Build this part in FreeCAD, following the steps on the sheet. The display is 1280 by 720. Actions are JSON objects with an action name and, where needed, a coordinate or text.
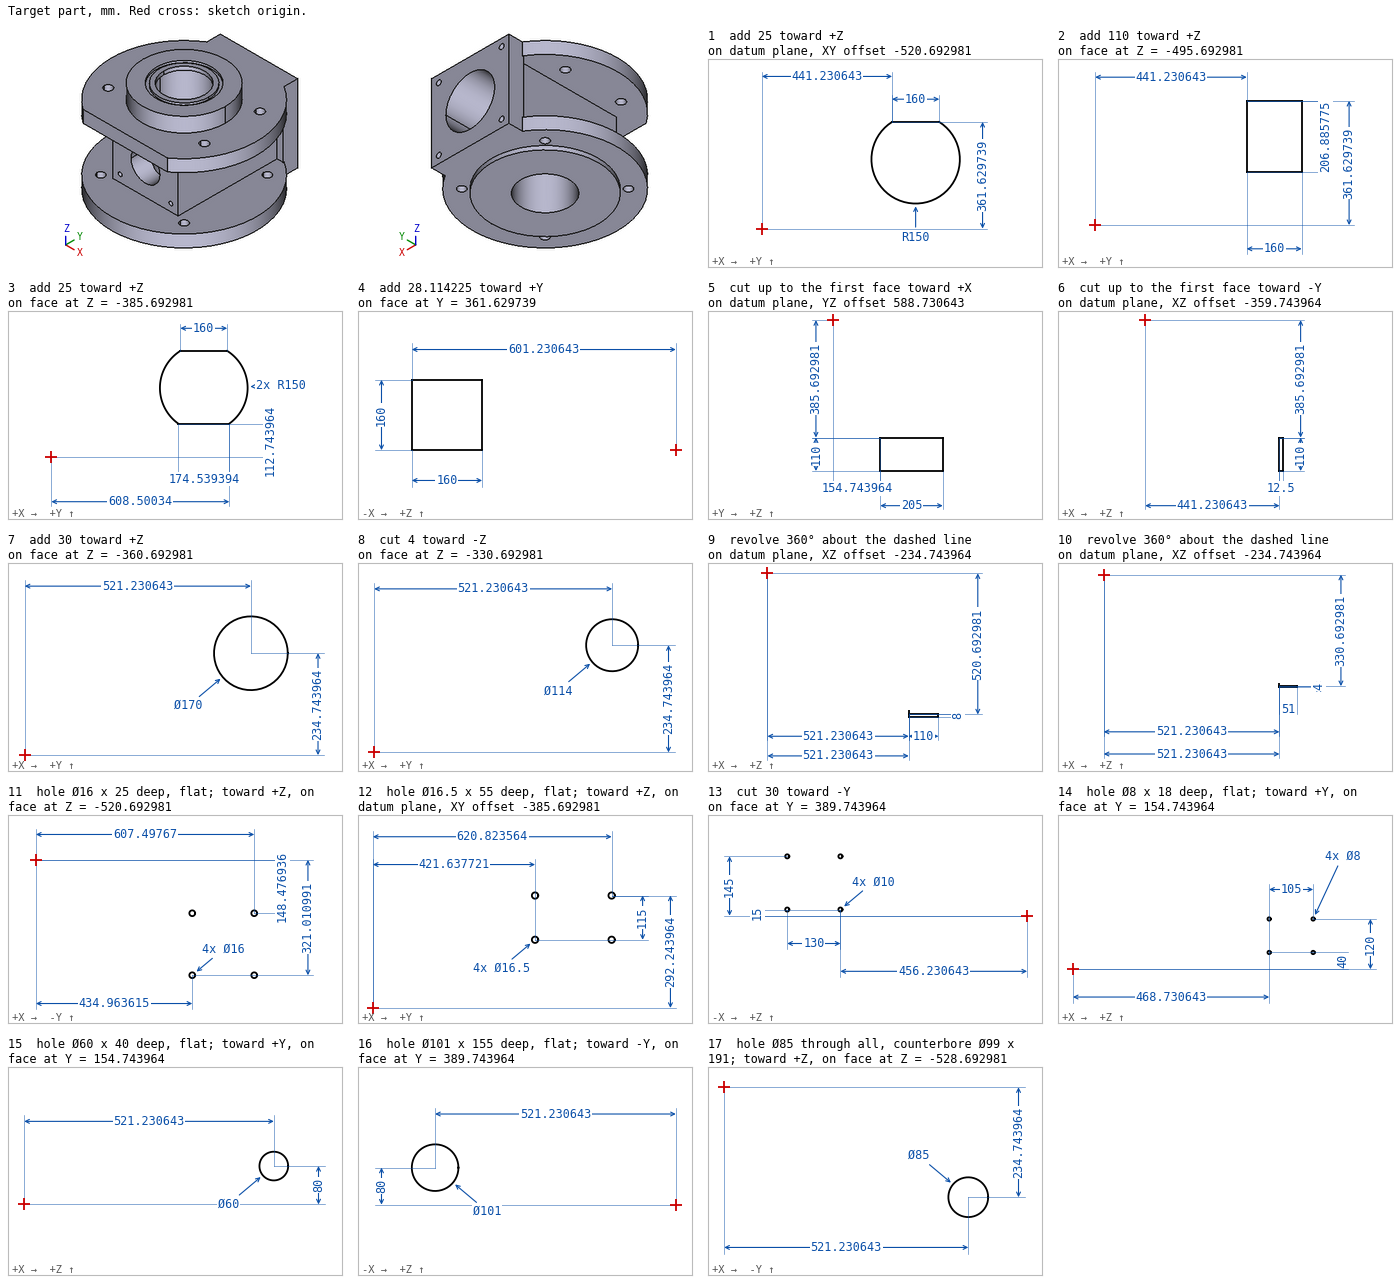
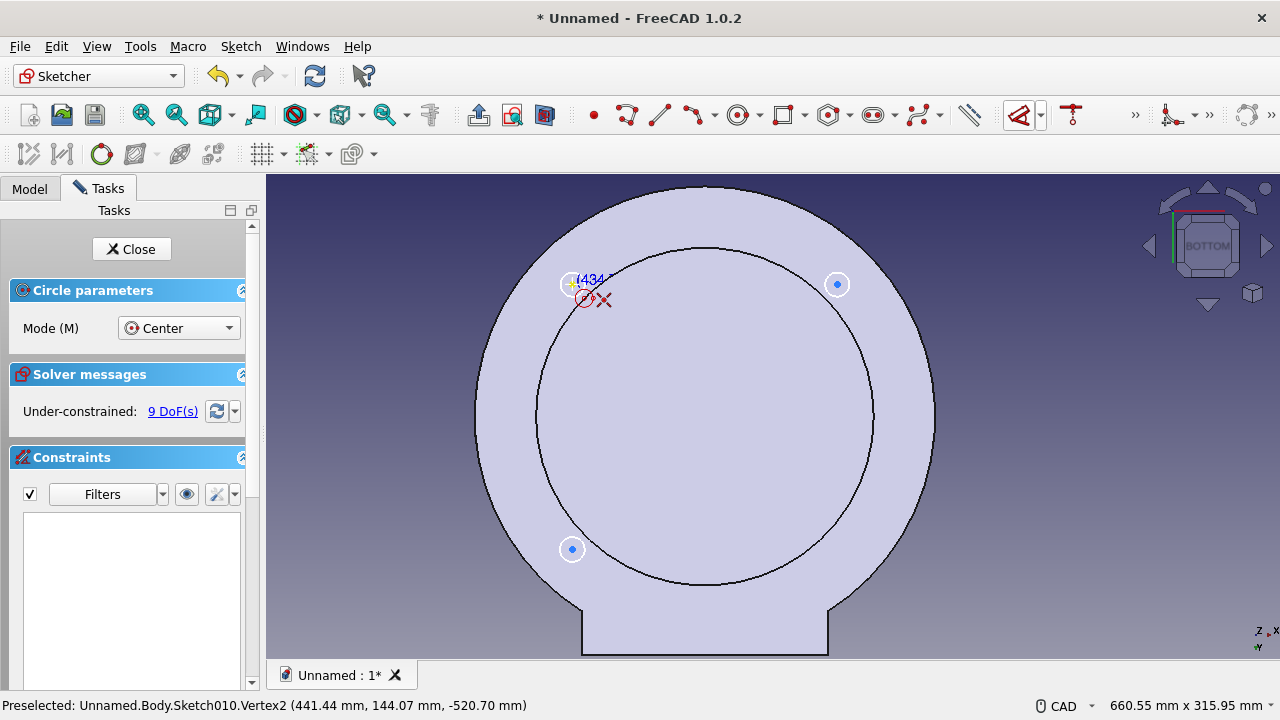
{"action": "scroll", "coordinate": [837, 549], "scroll_direction": "up", "scroll_amount": 4}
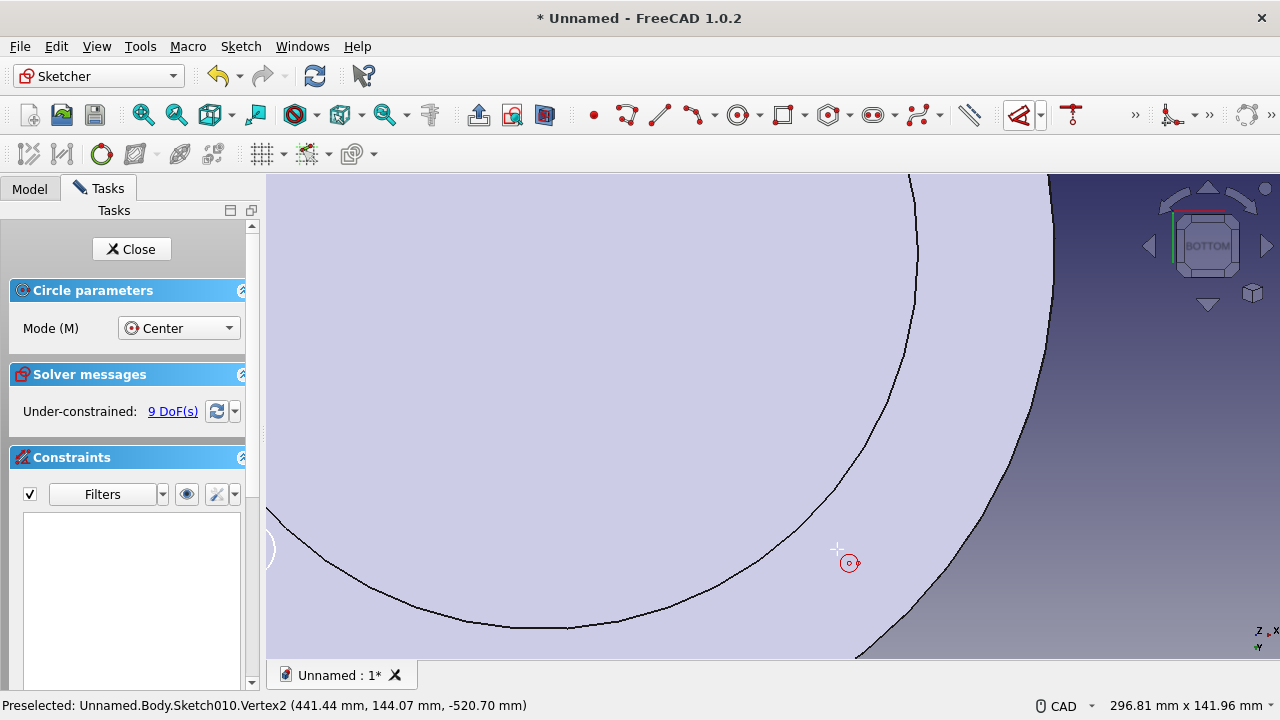
{"action": "left_click", "coordinate": [837, 548]}
{"action": "left_click", "coordinate": [856, 529]}
{"action": "key", "text": "Escape"}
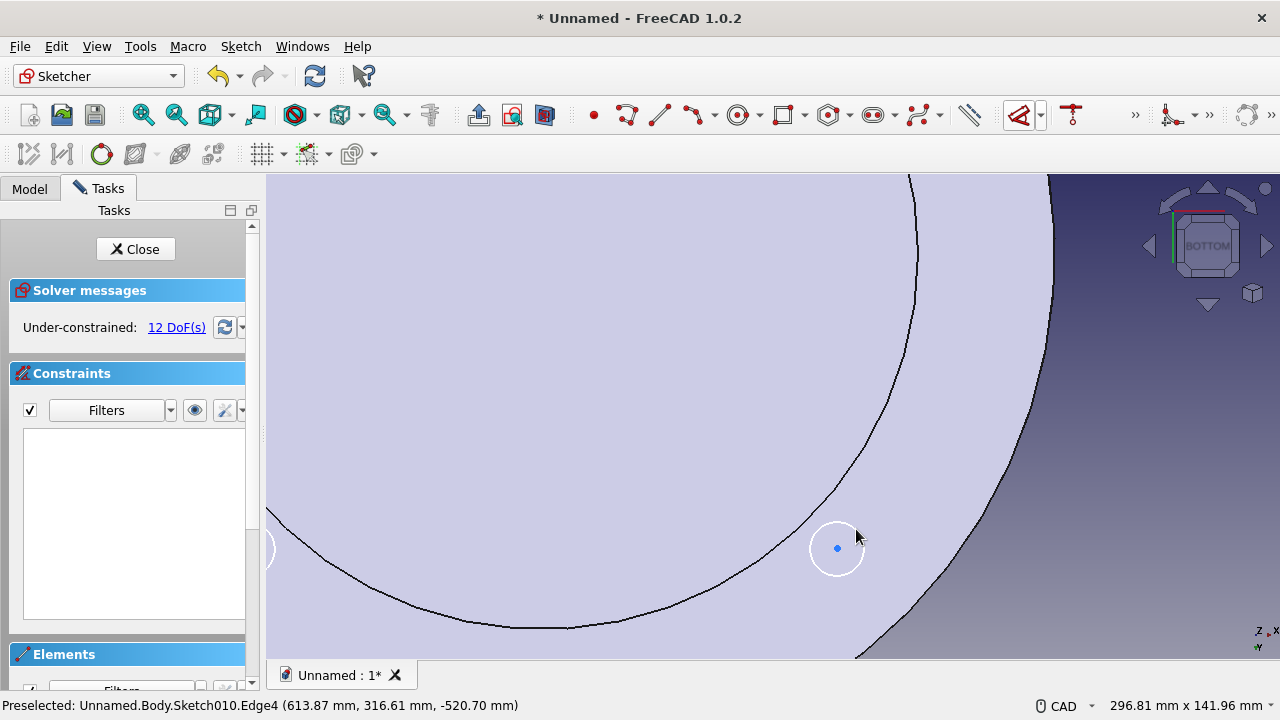
{"action": "scroll", "coordinate": [837, 549], "scroll_direction": "down", "scroll_amount": 4}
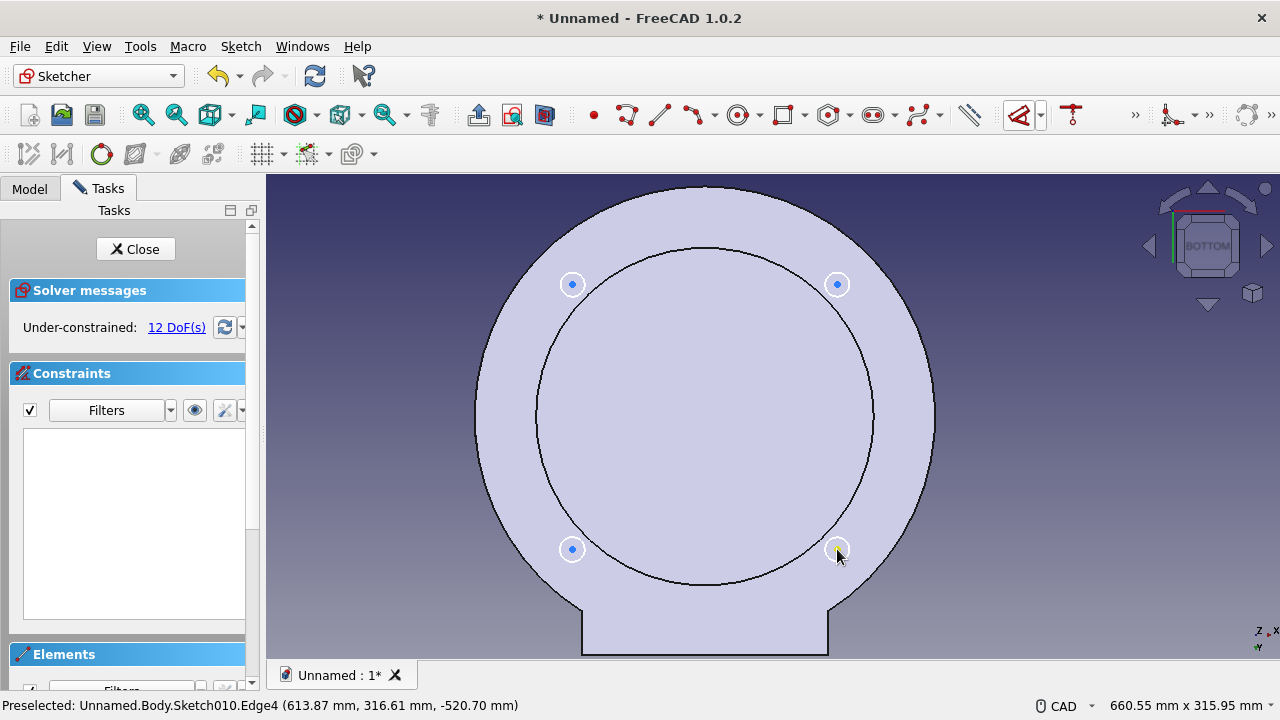
{"action": "left_click", "coordinate": [581, 541]}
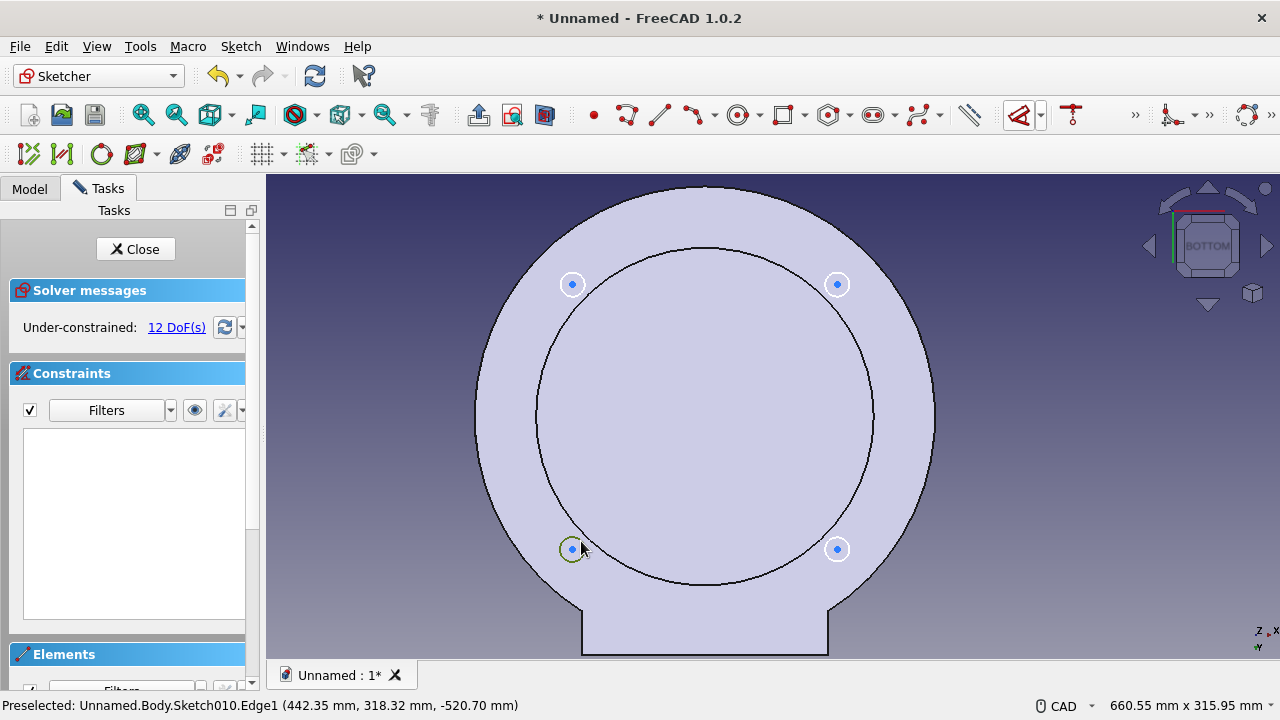
{"action": "left_click", "coordinate": [846, 276]}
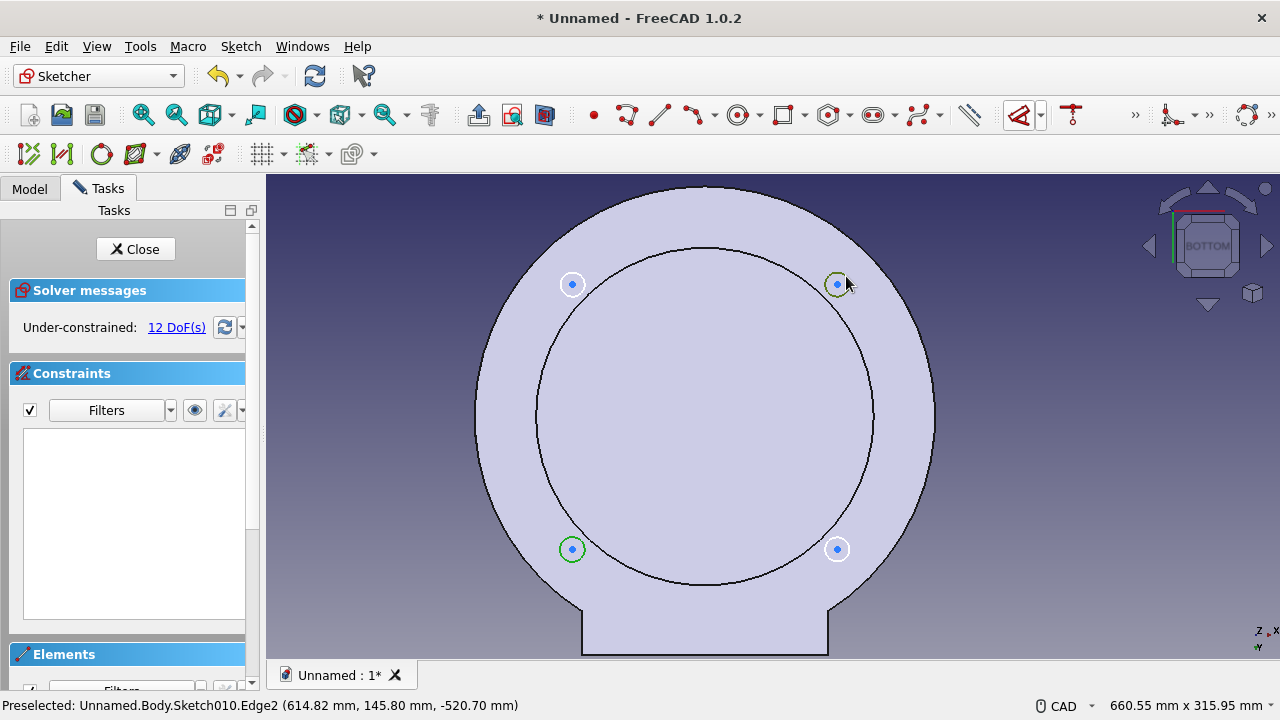
{"action": "left_click", "coordinate": [581, 276]}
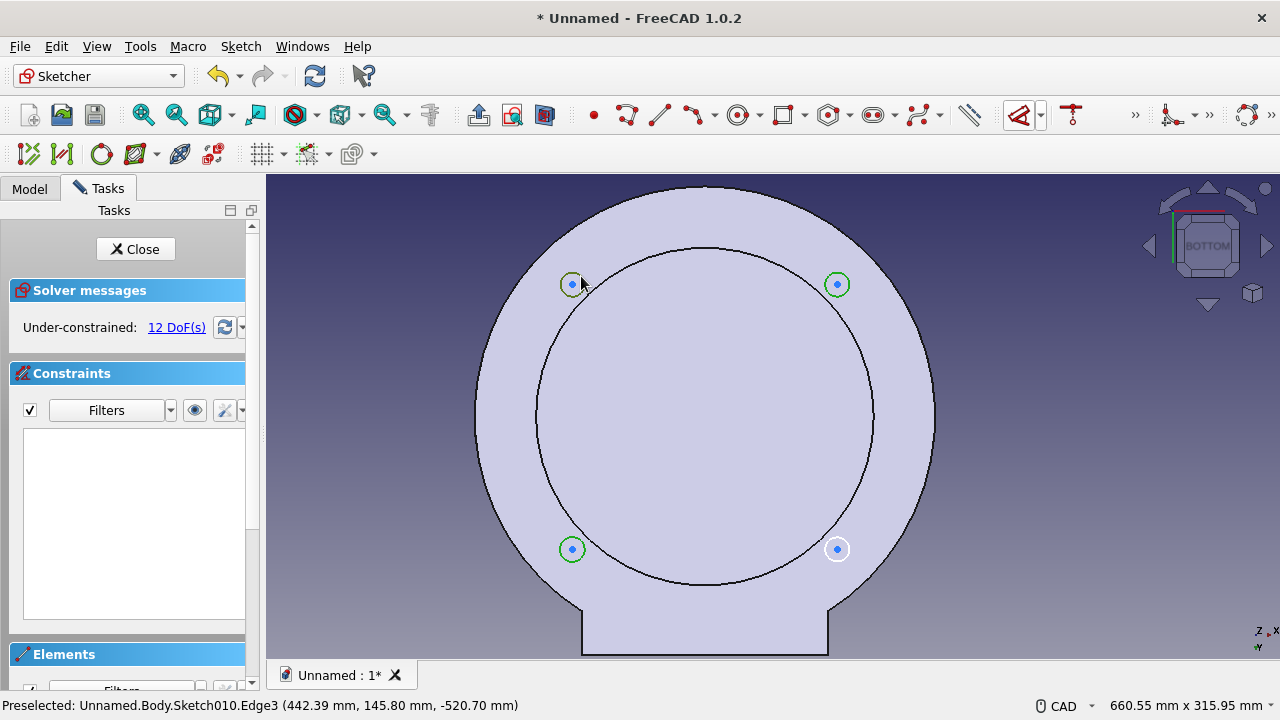
{"action": "left_click", "coordinate": [846, 541]}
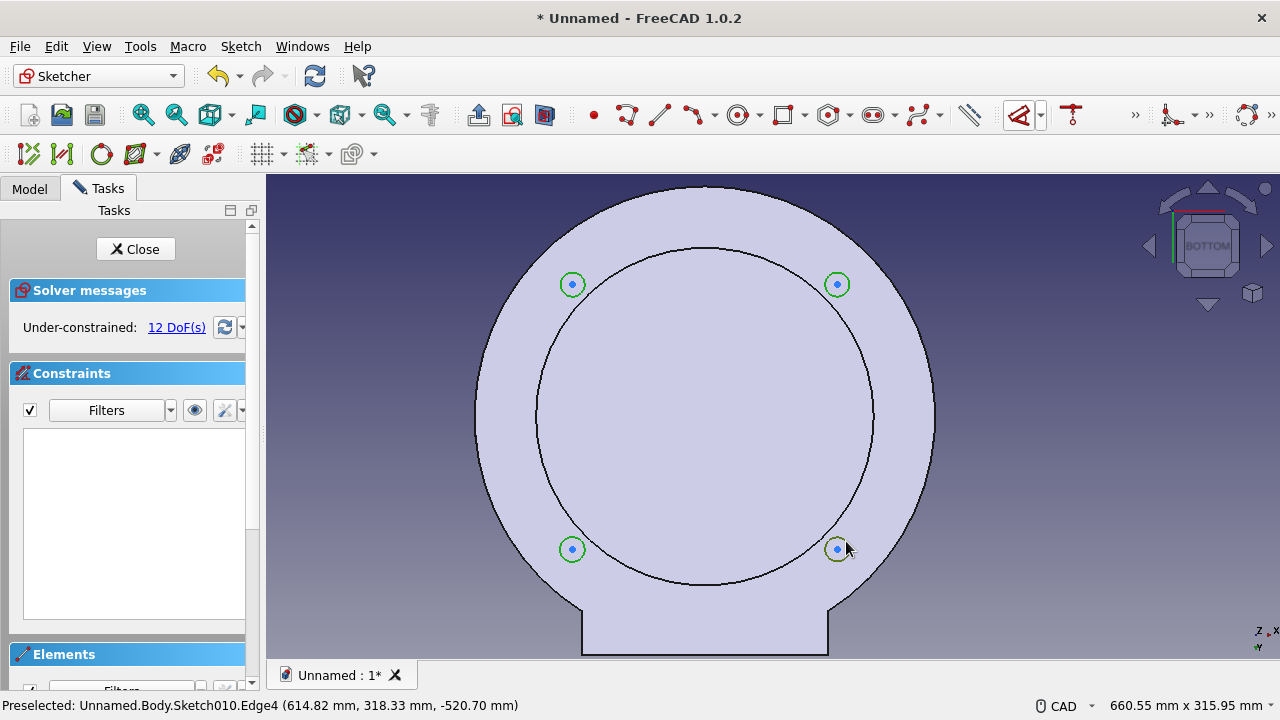
{"action": "key", "text": "e"}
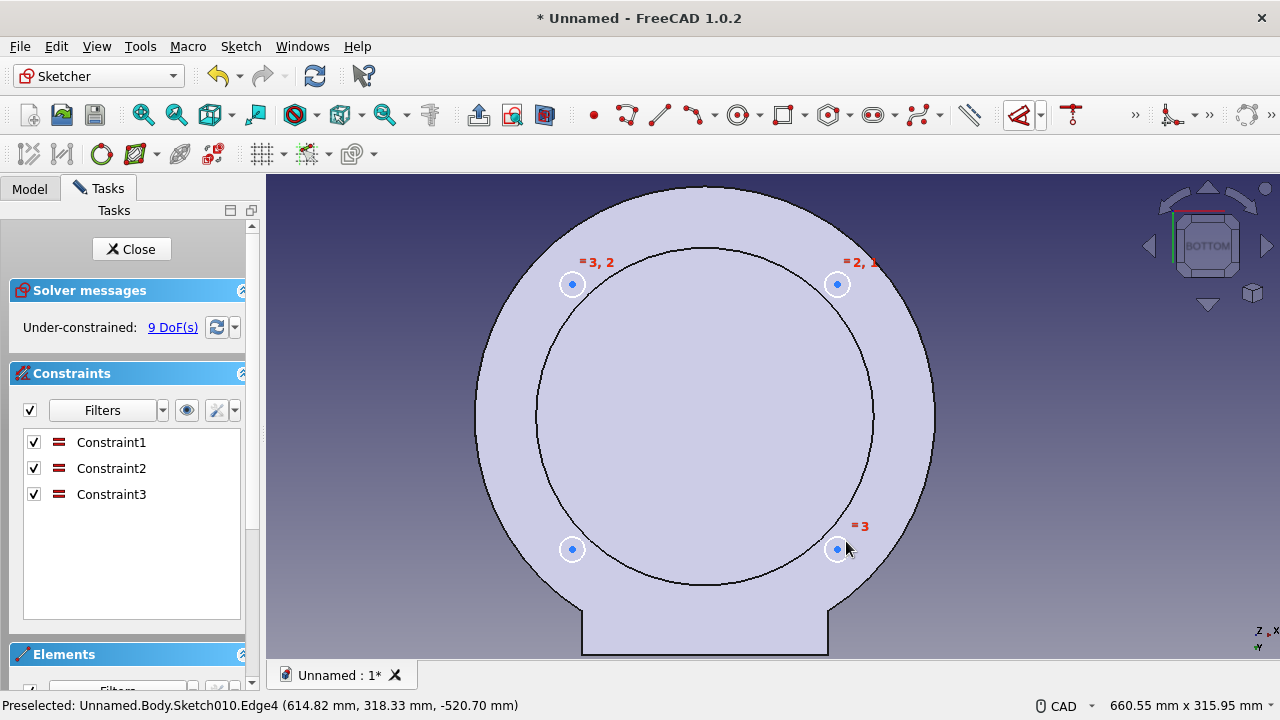
{"action": "left_click", "coordinate": [572, 550]}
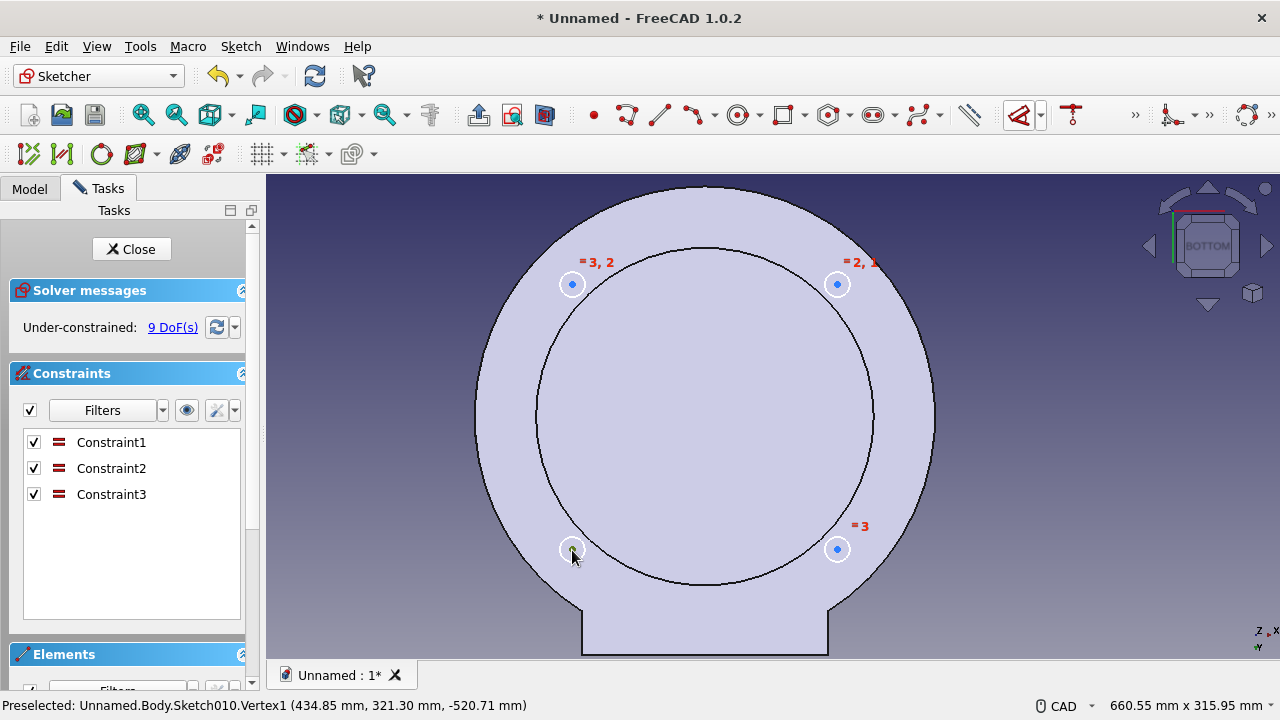
{"action": "left_click", "coordinate": [573, 285]}